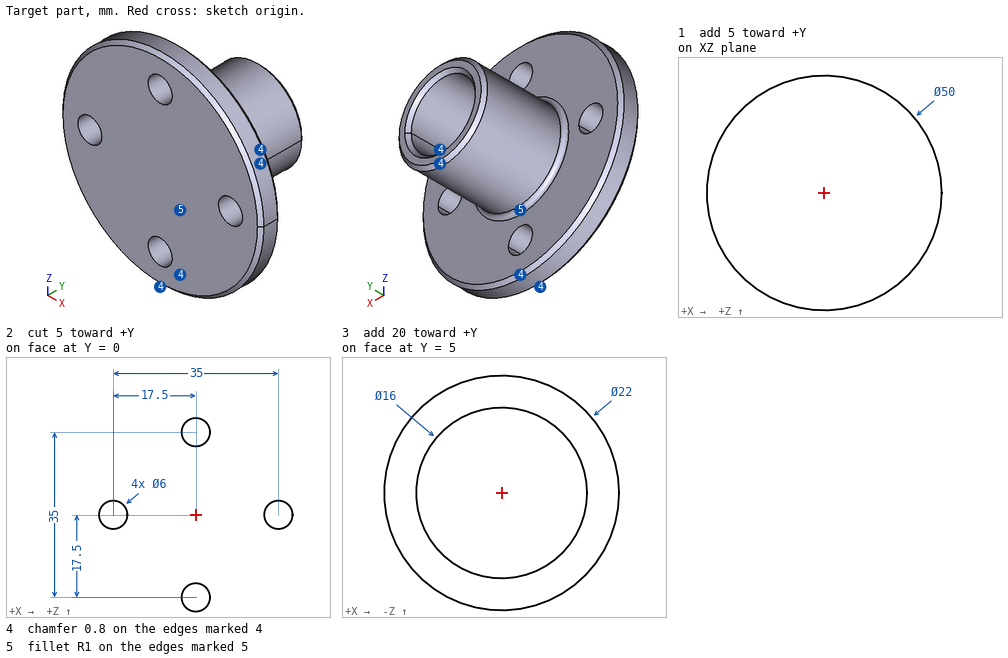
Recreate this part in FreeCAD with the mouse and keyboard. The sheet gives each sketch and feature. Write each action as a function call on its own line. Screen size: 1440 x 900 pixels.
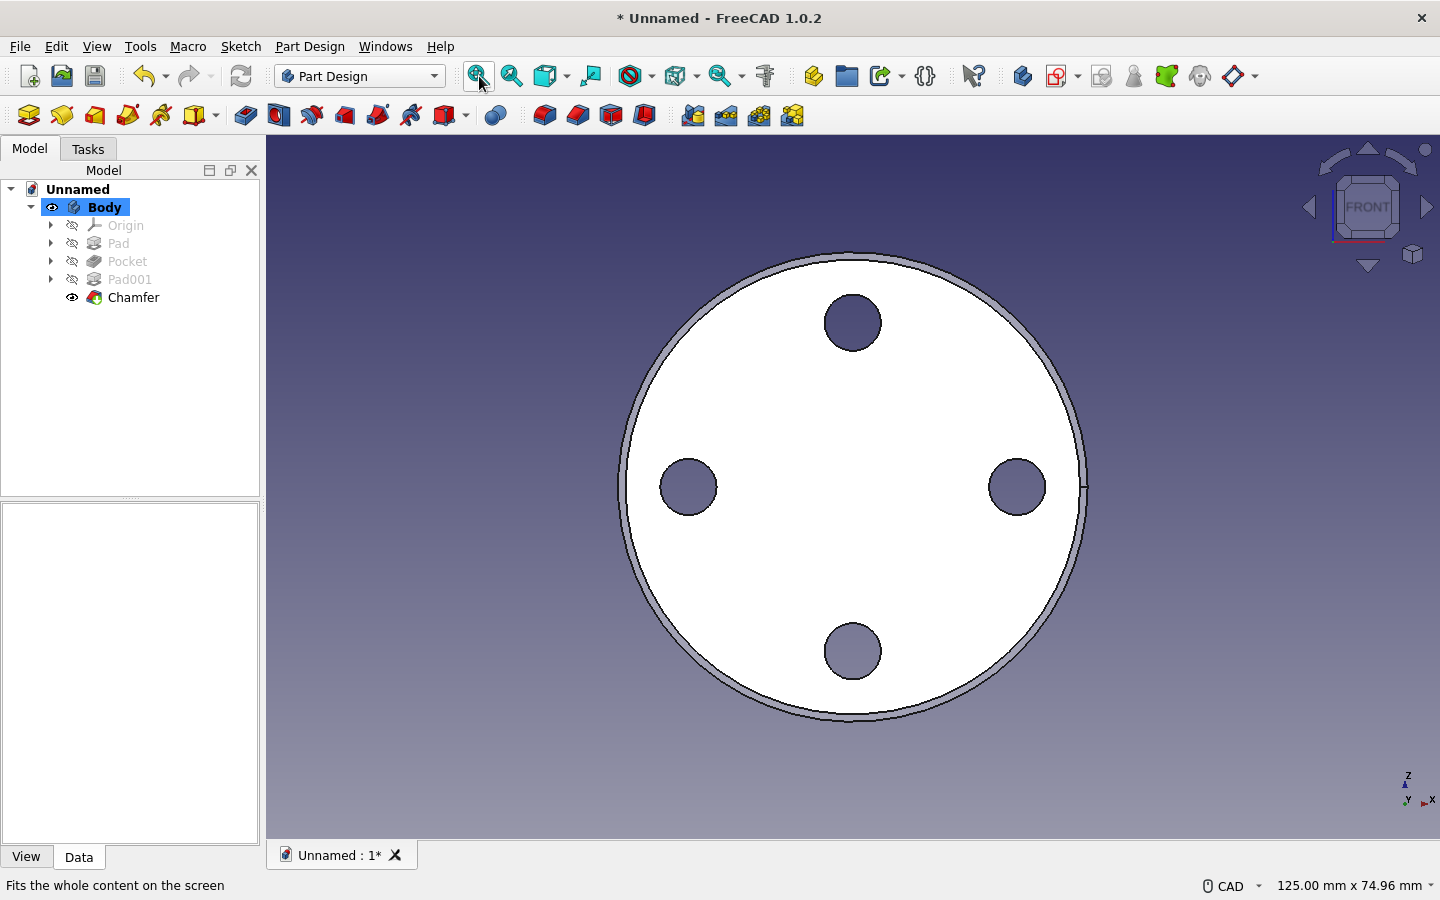
key(3)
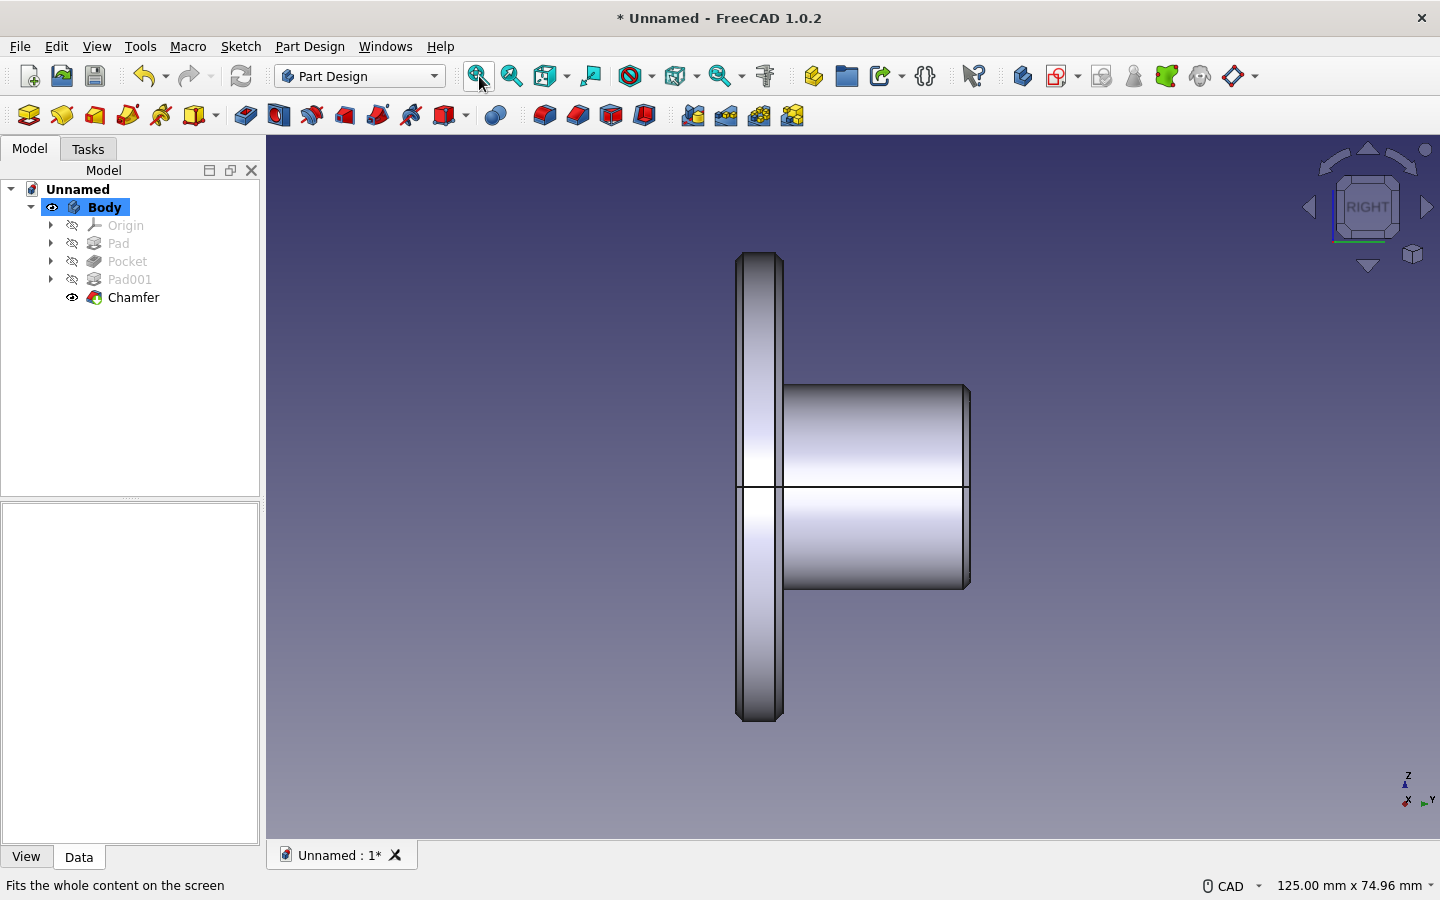
key(5)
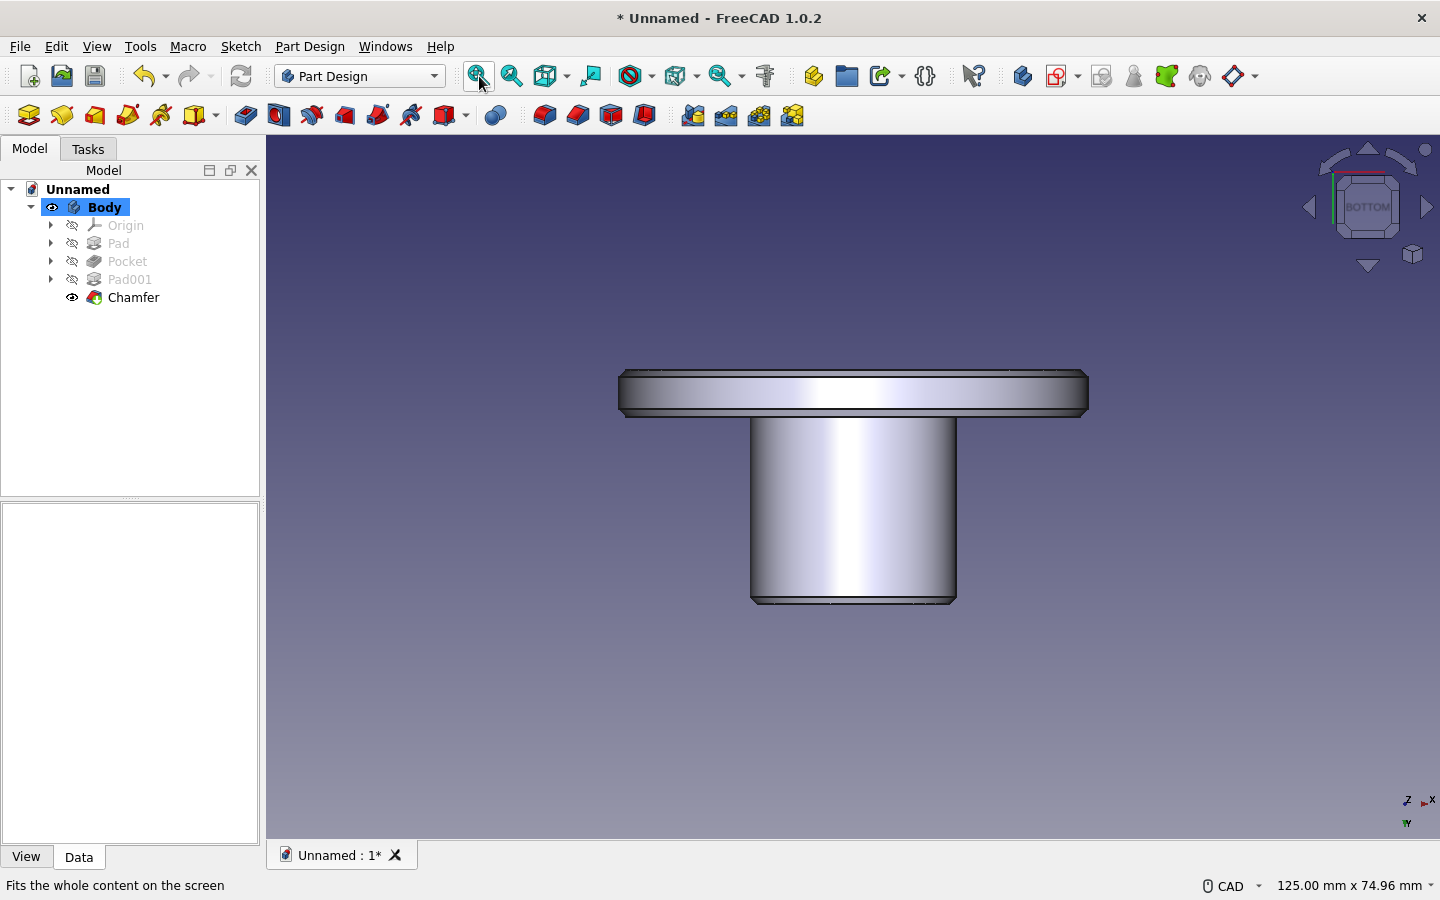
click(479, 76)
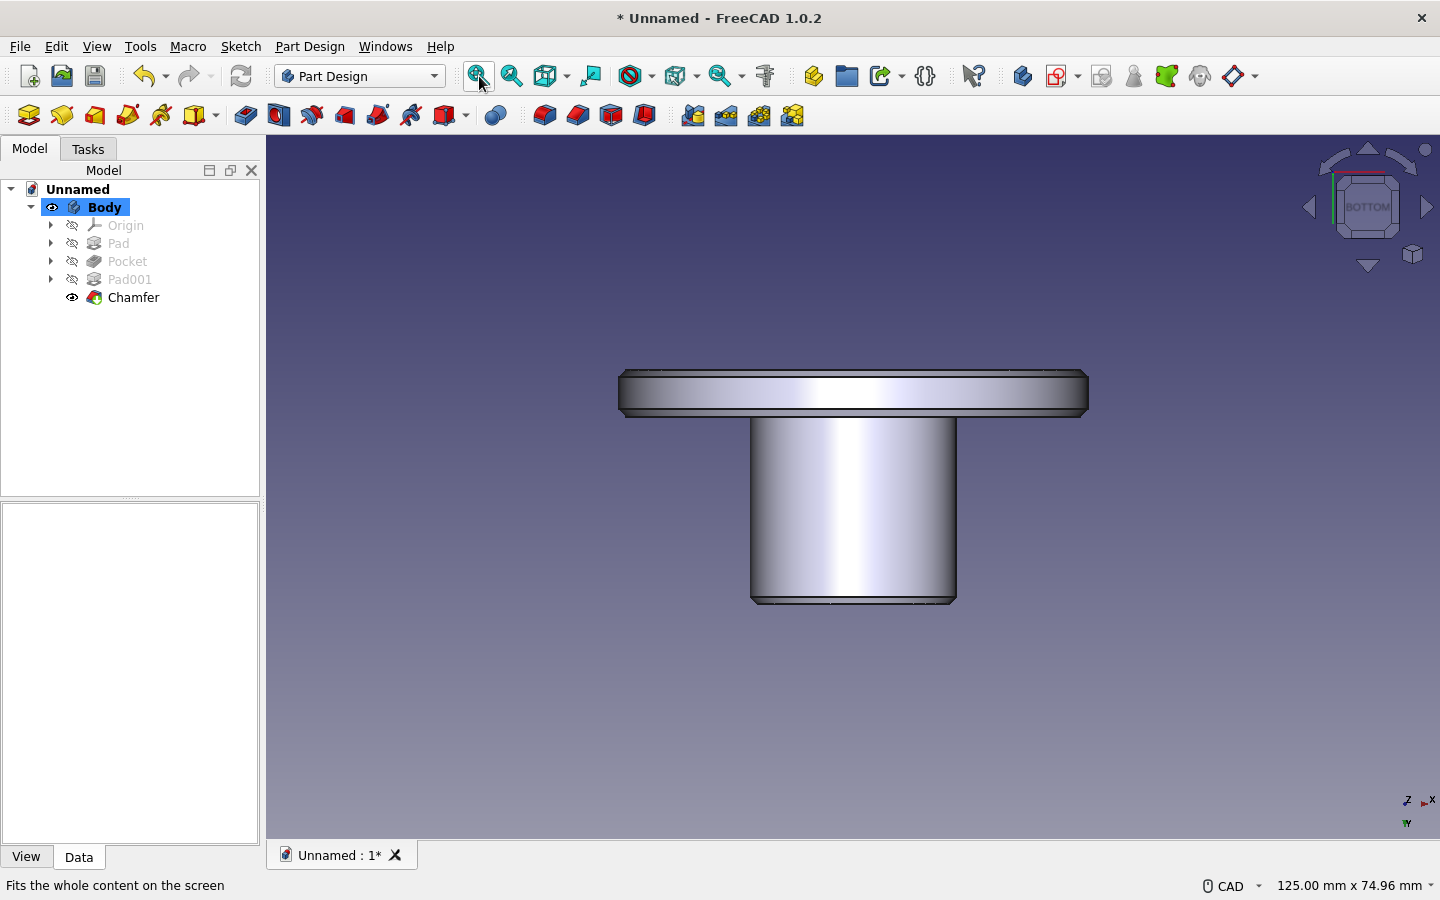
key(4)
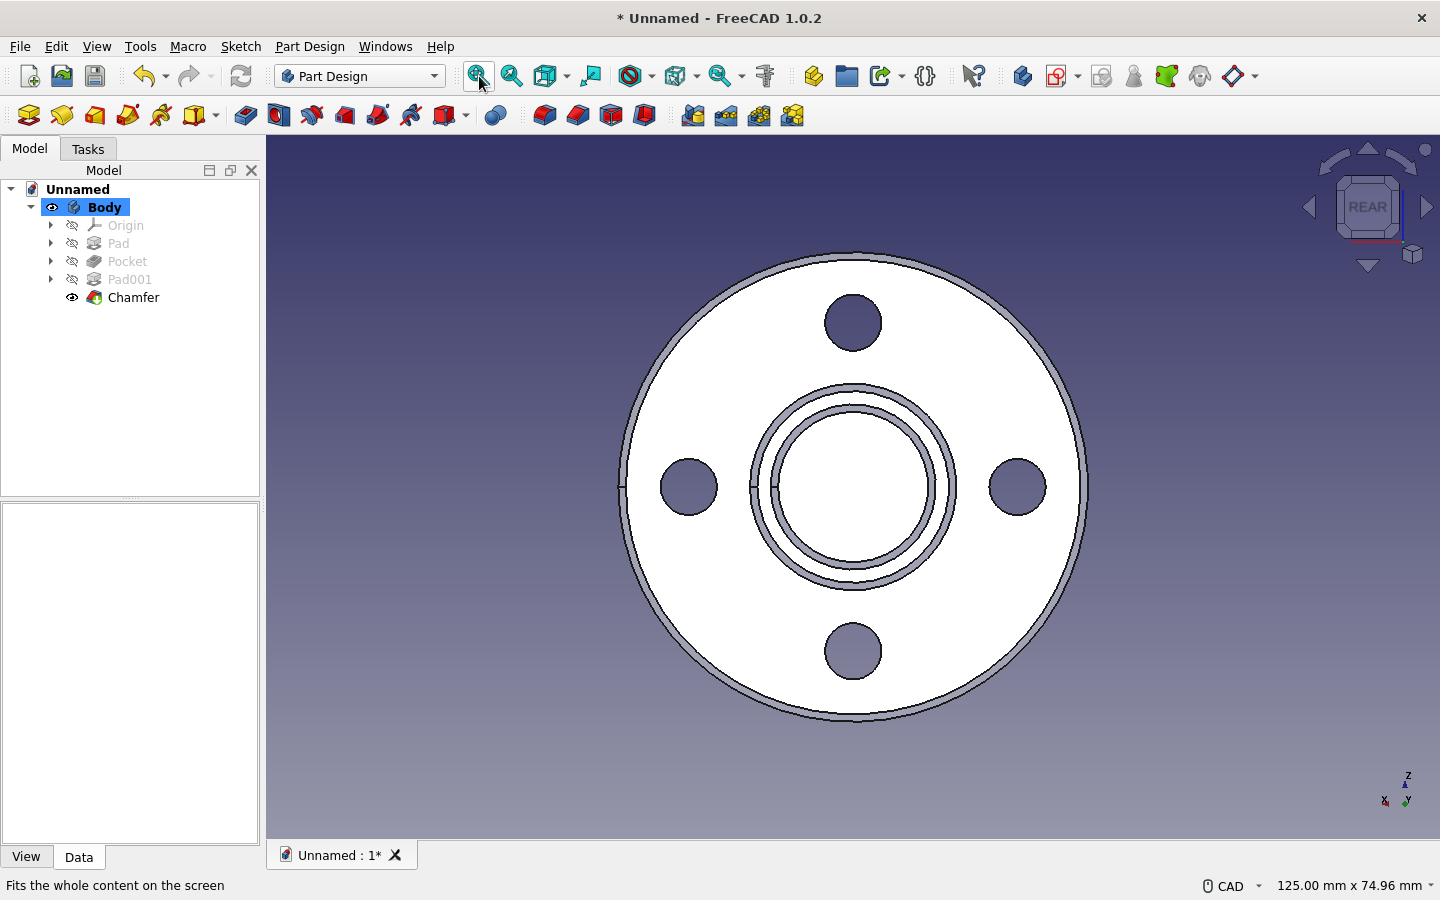
key(6)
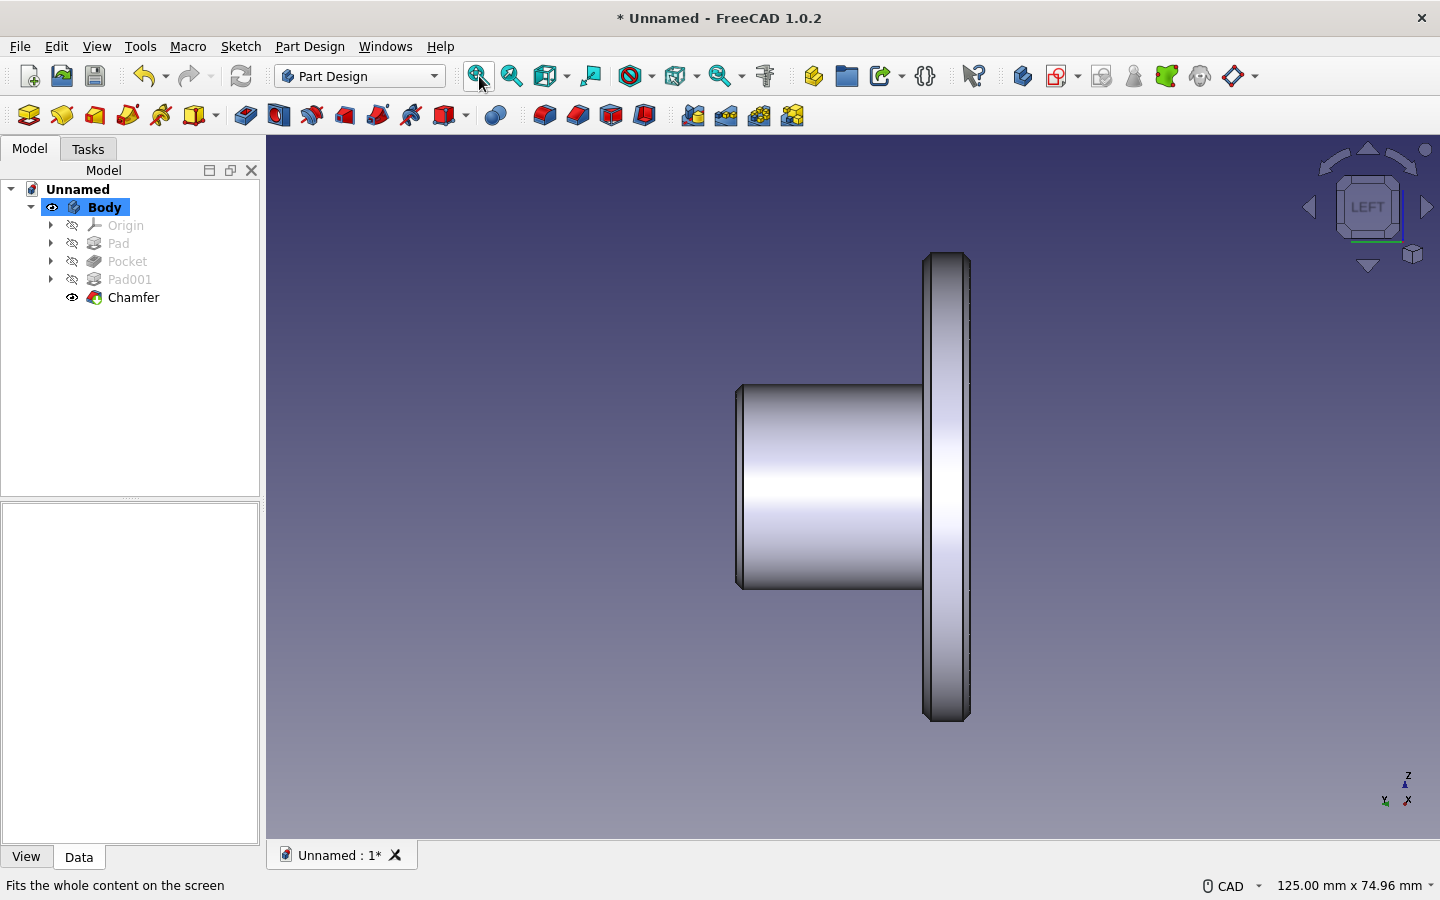
key(v)
key(3)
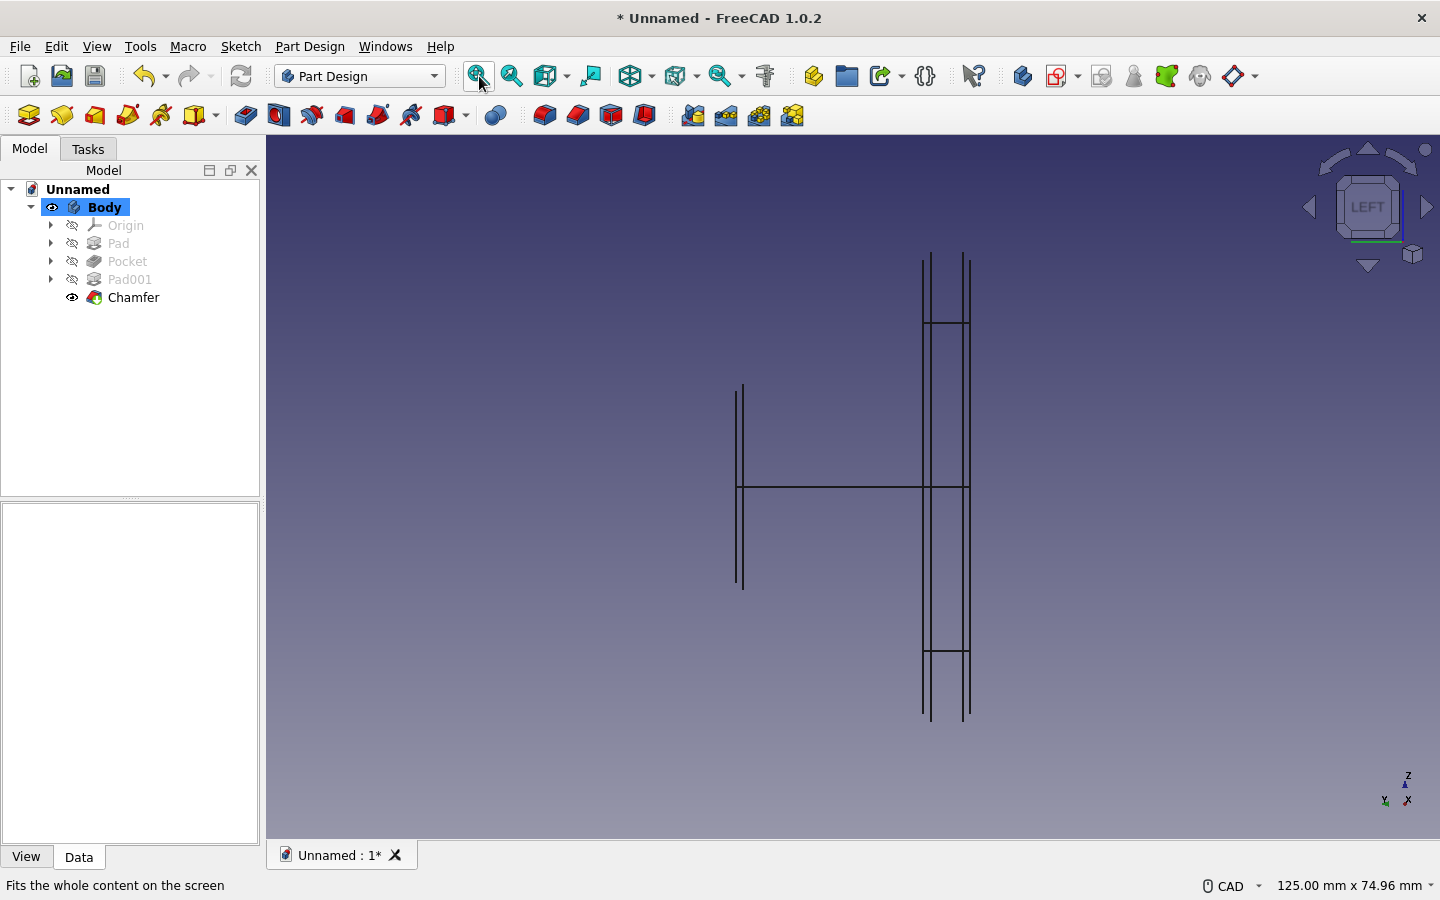
key(0)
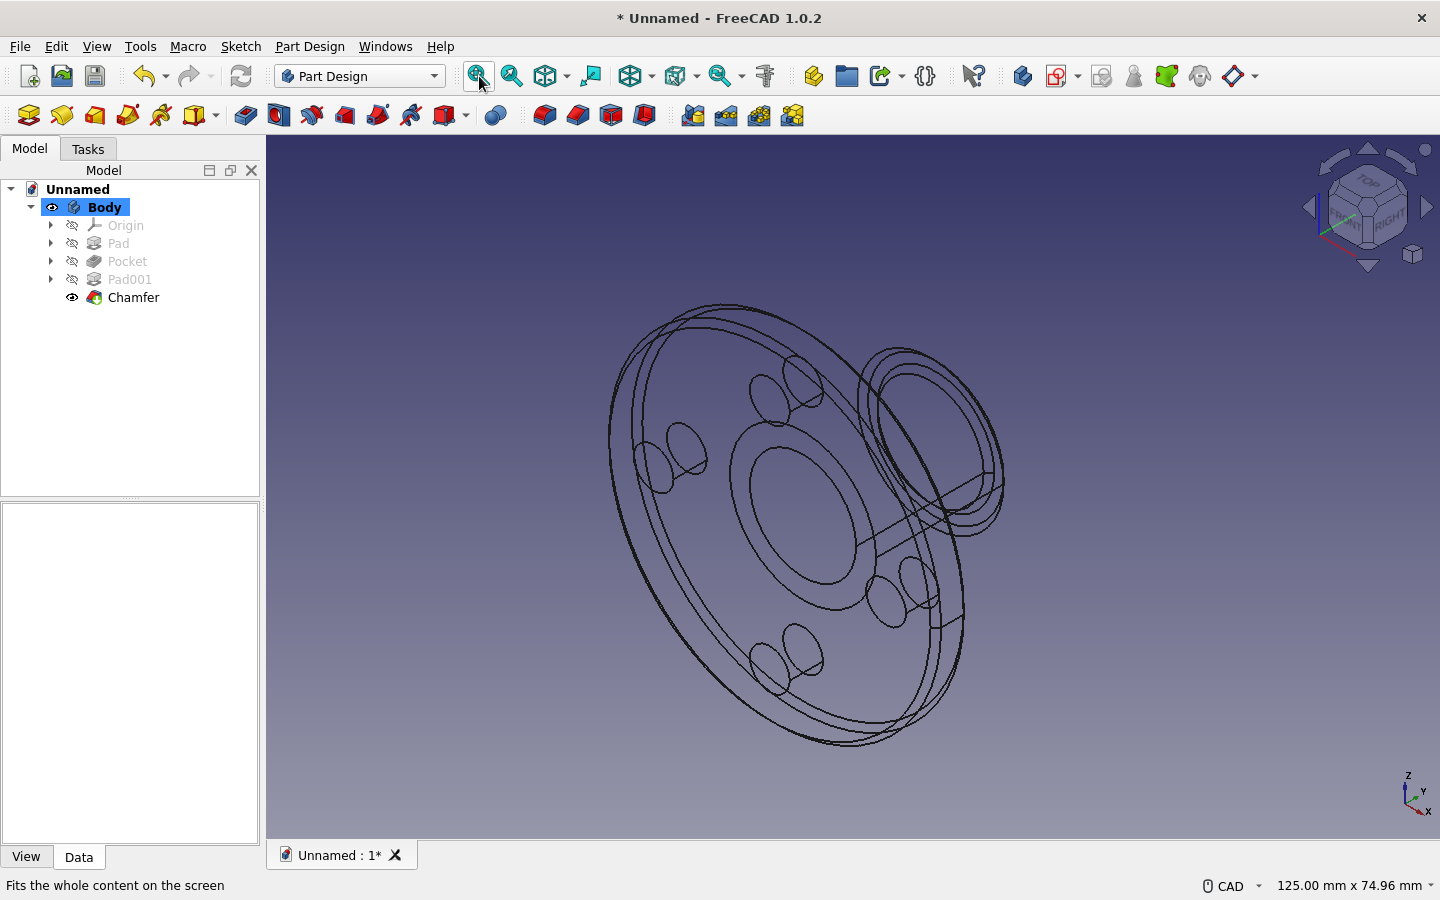
click(730, 473)